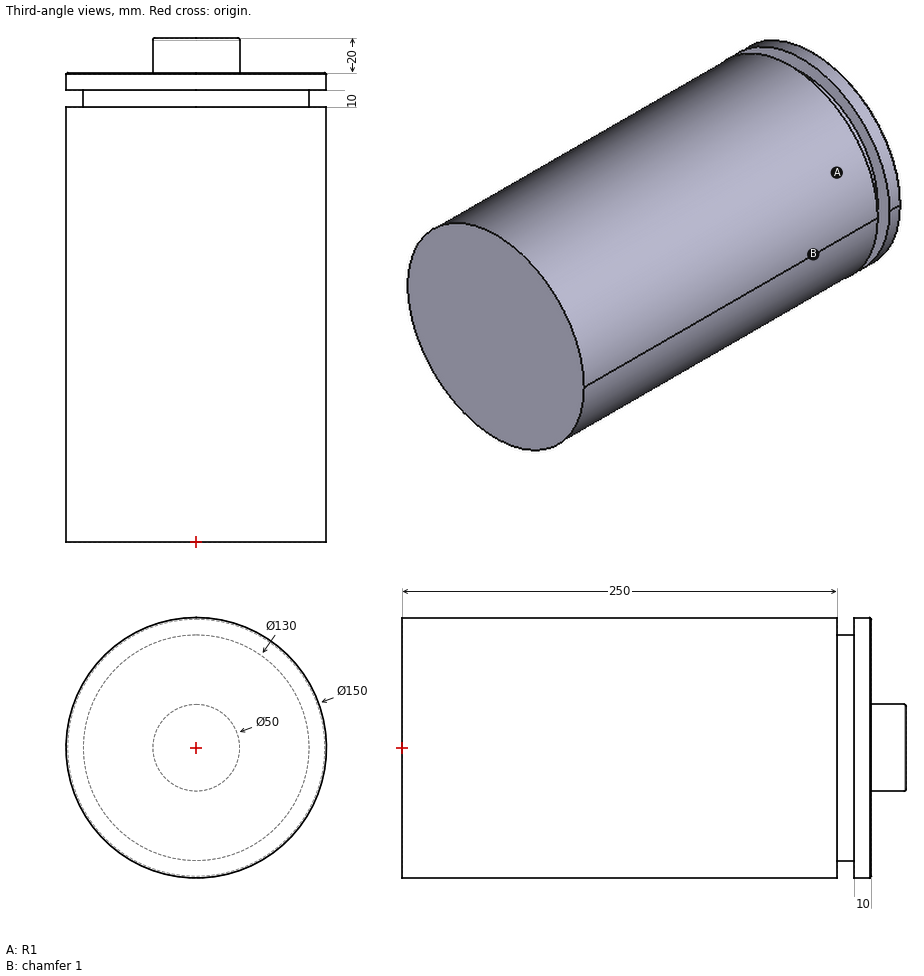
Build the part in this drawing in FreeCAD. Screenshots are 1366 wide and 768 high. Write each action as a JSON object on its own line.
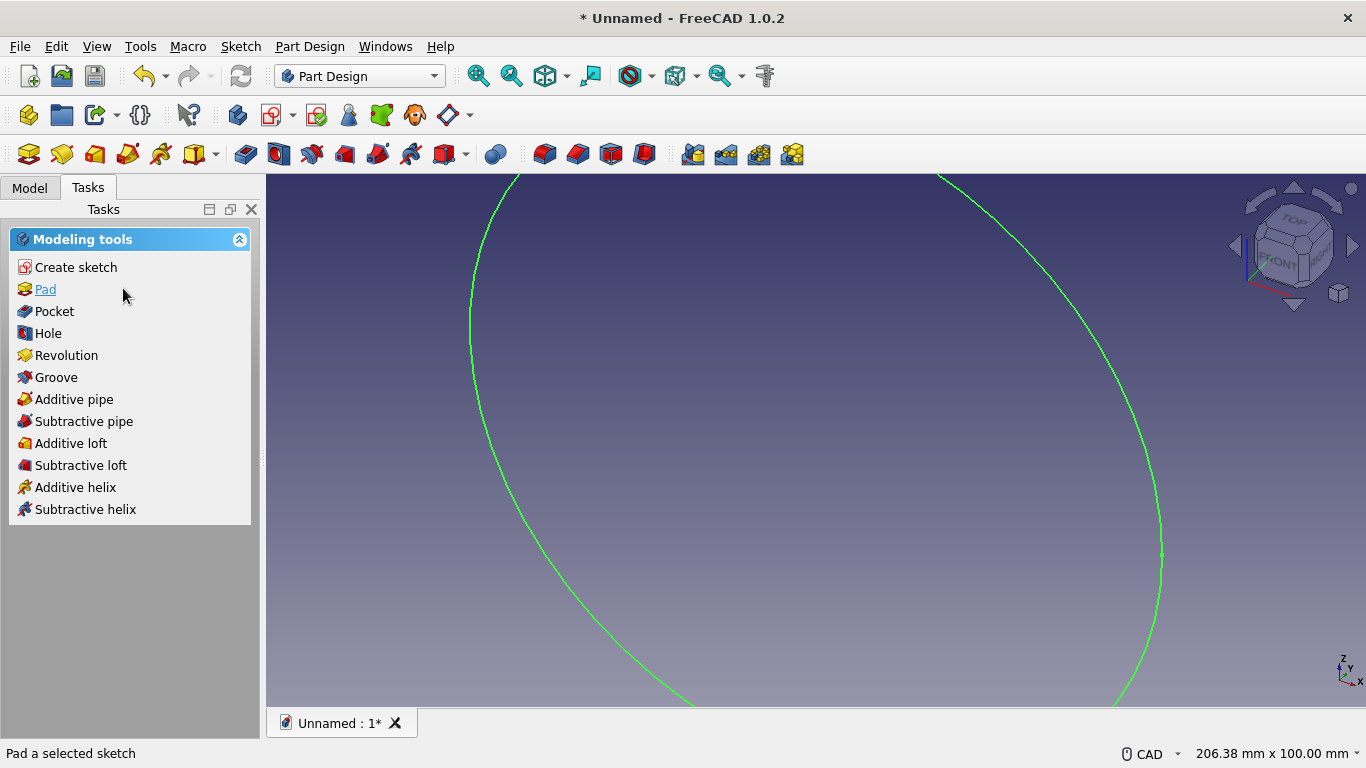
{"action": "left_click", "coordinate": [29, 154]}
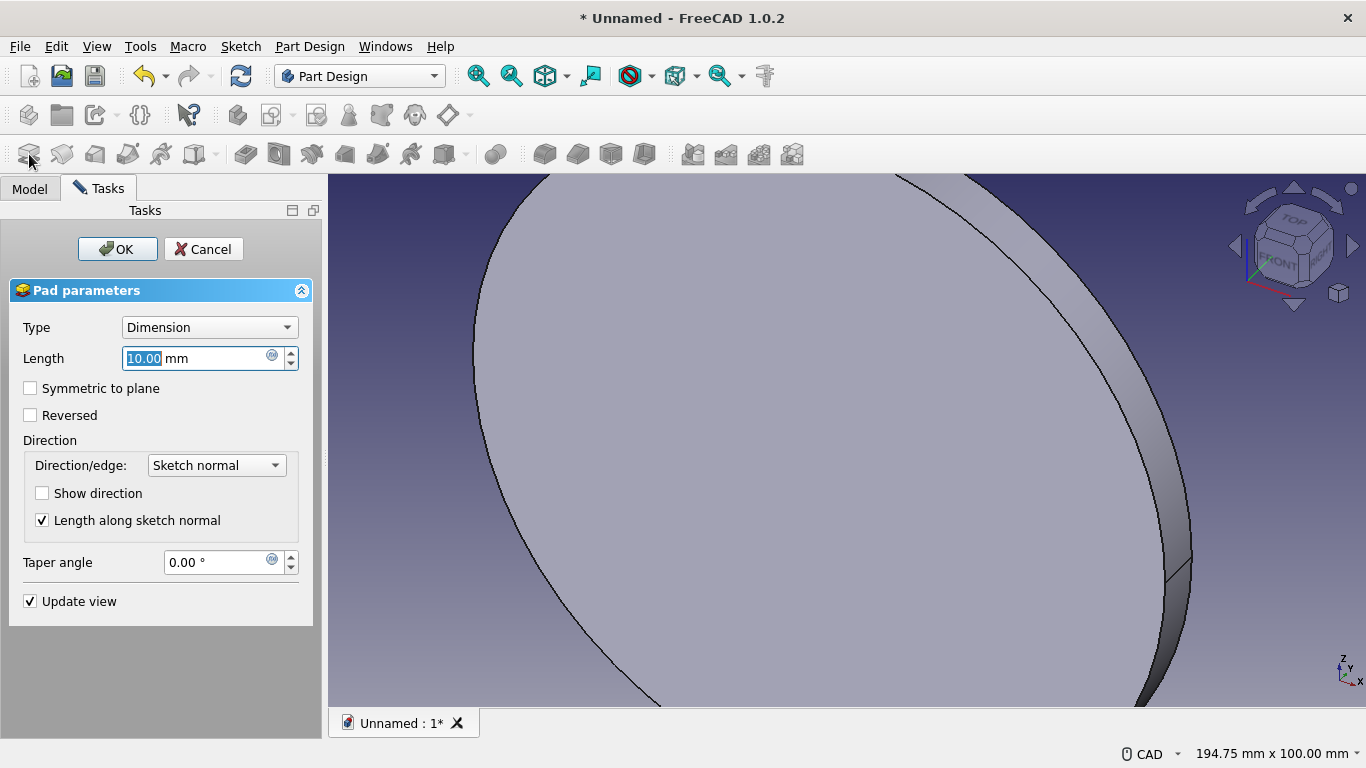
{"action": "type", "text": "250"}
{"action": "key", "text": "Tab"}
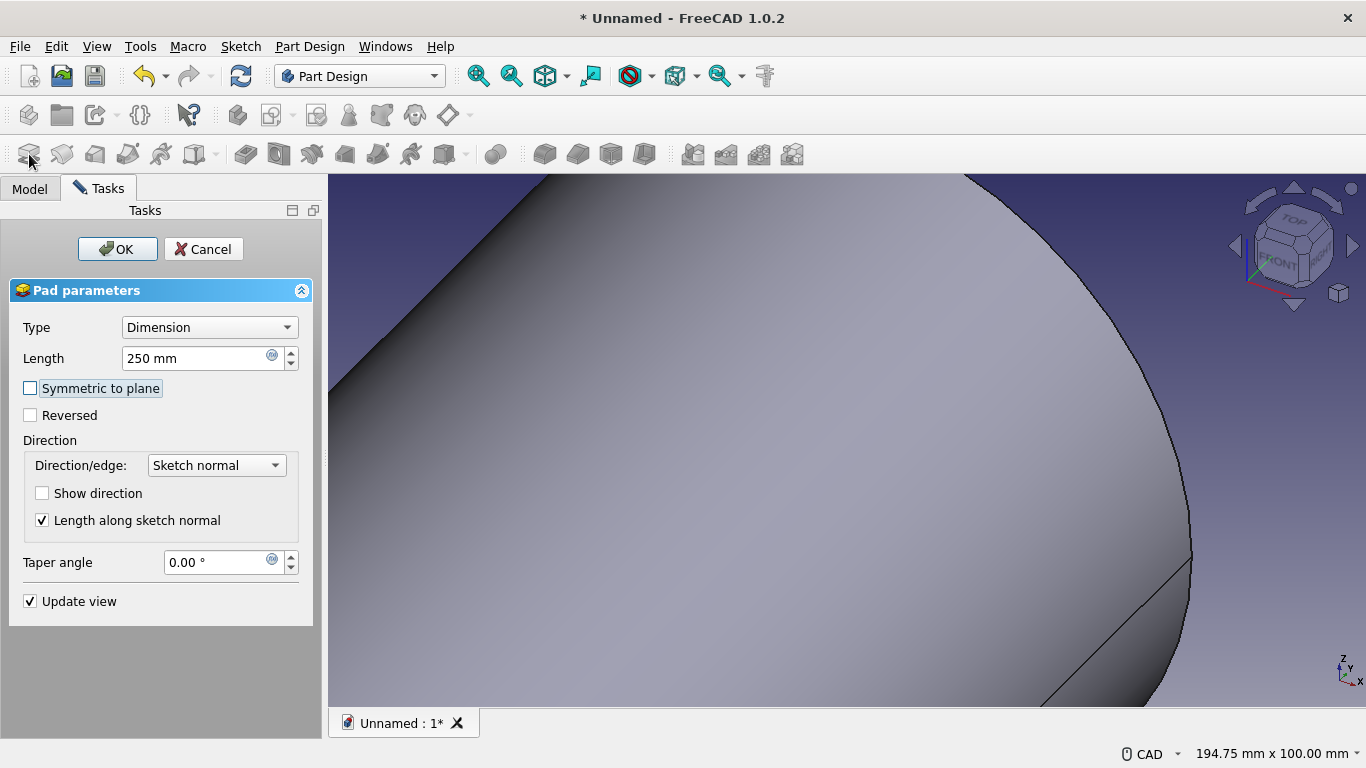
{"action": "left_click", "coordinate": [31, 415]}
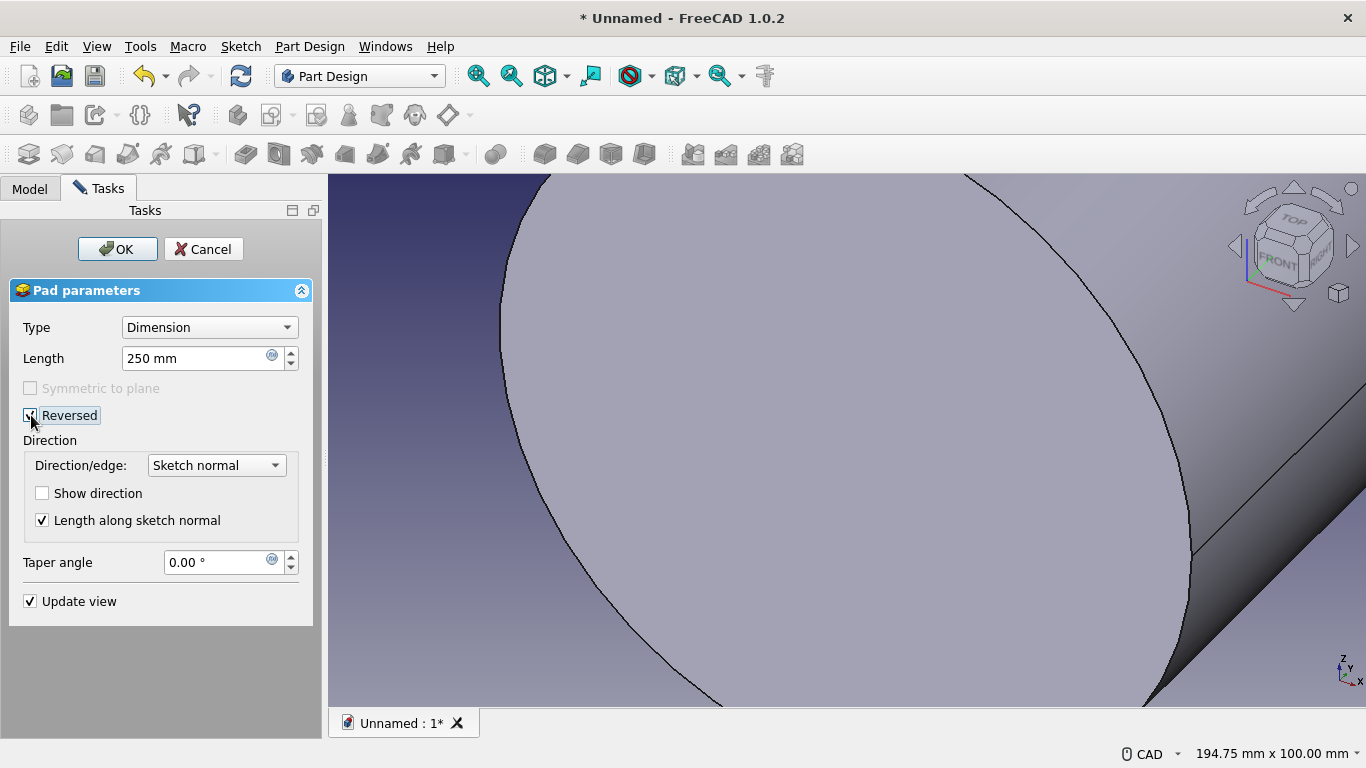
{"action": "left_click", "coordinate": [118, 249]}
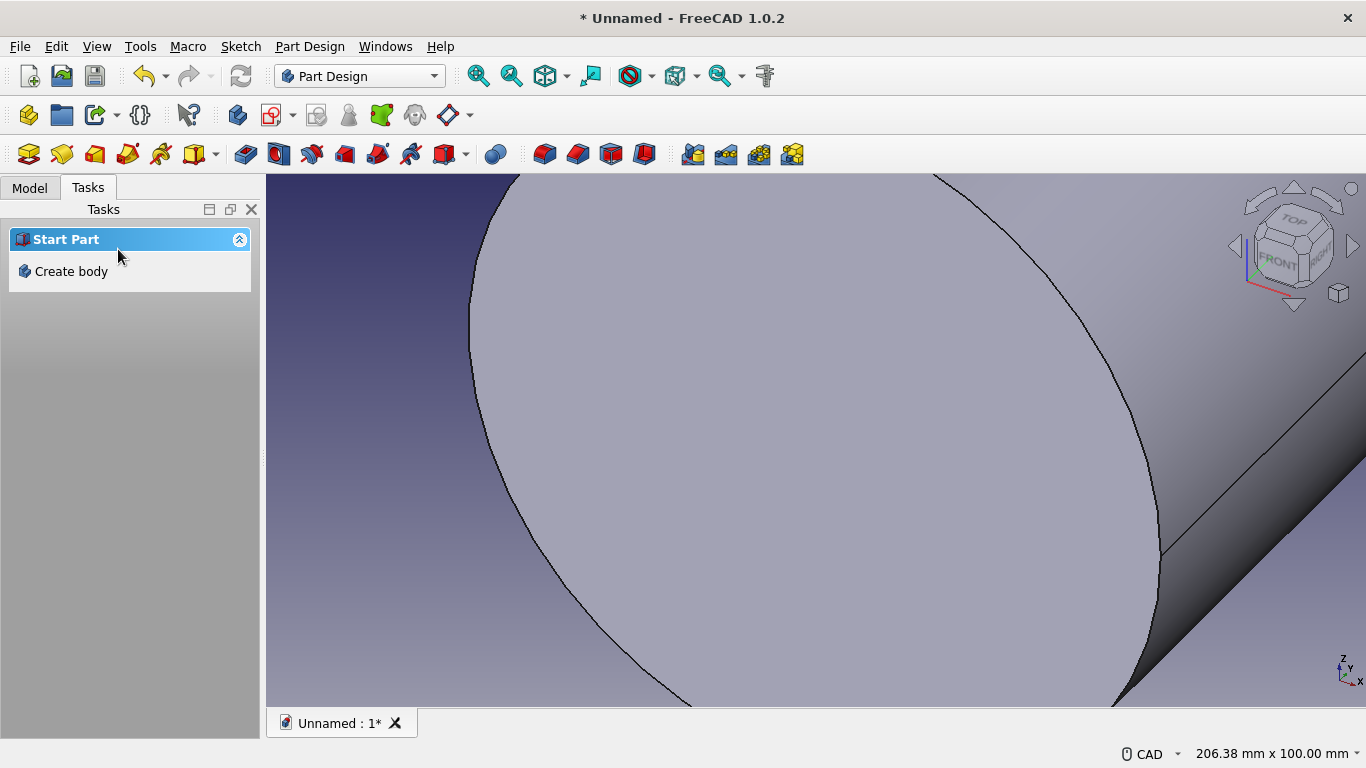
{"action": "key", "text": "v f"}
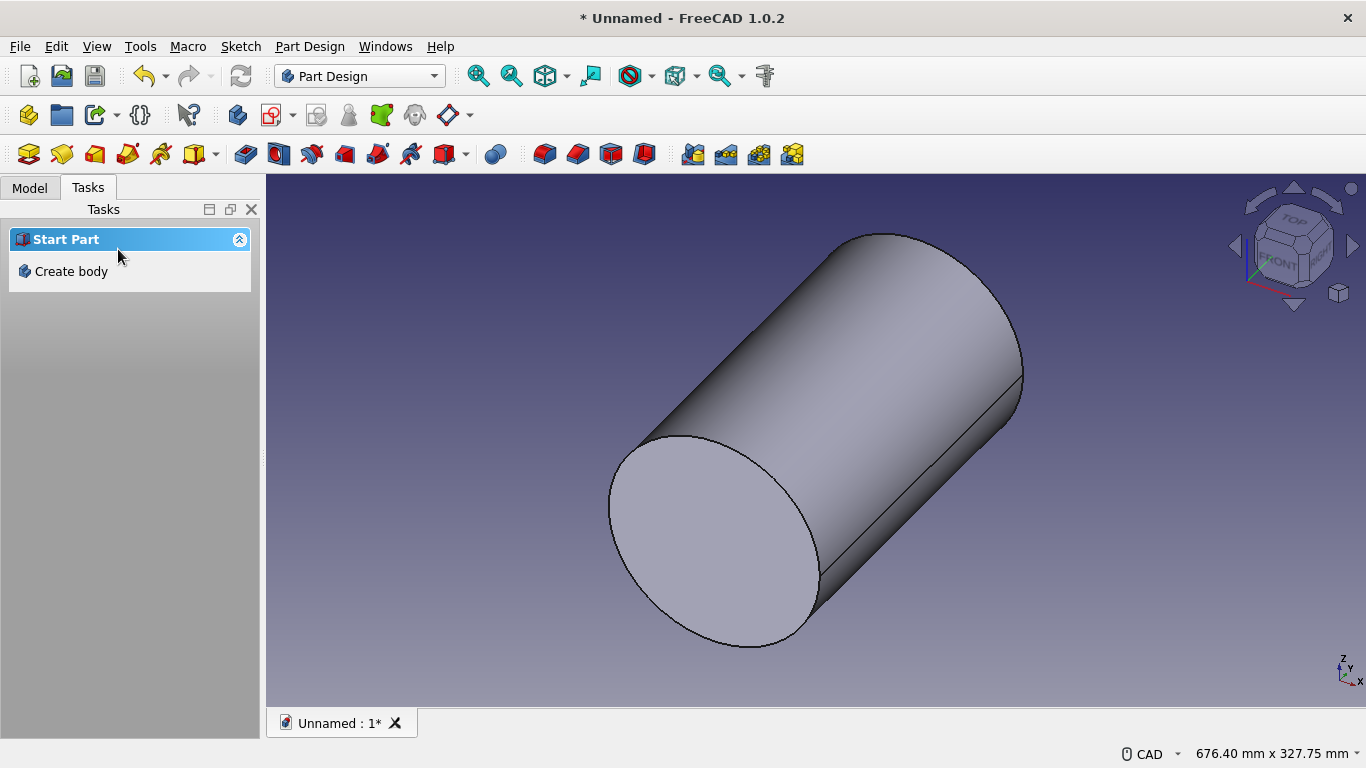
{"action": "key", "text": "4"}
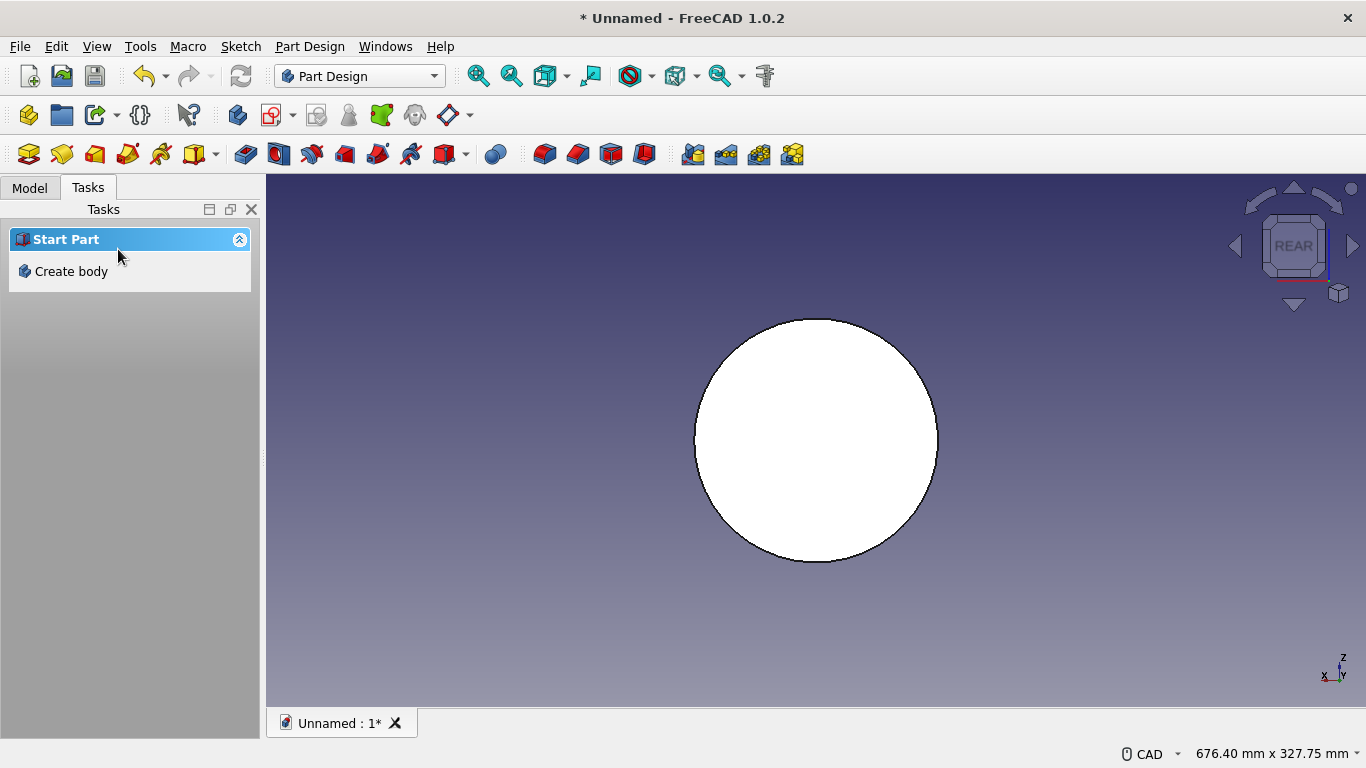
{"action": "left_click", "coordinate": [816, 440]}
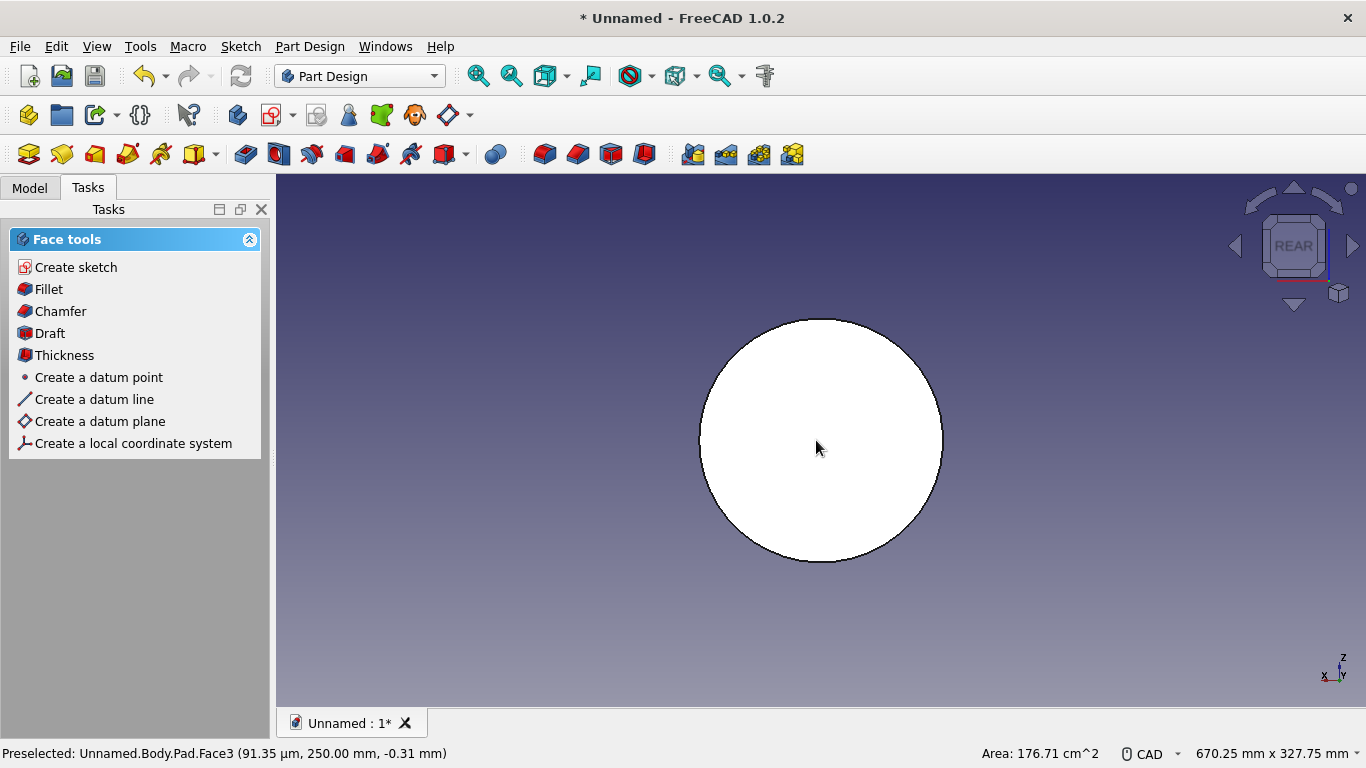
{"action": "left_click", "coordinate": [270, 116]}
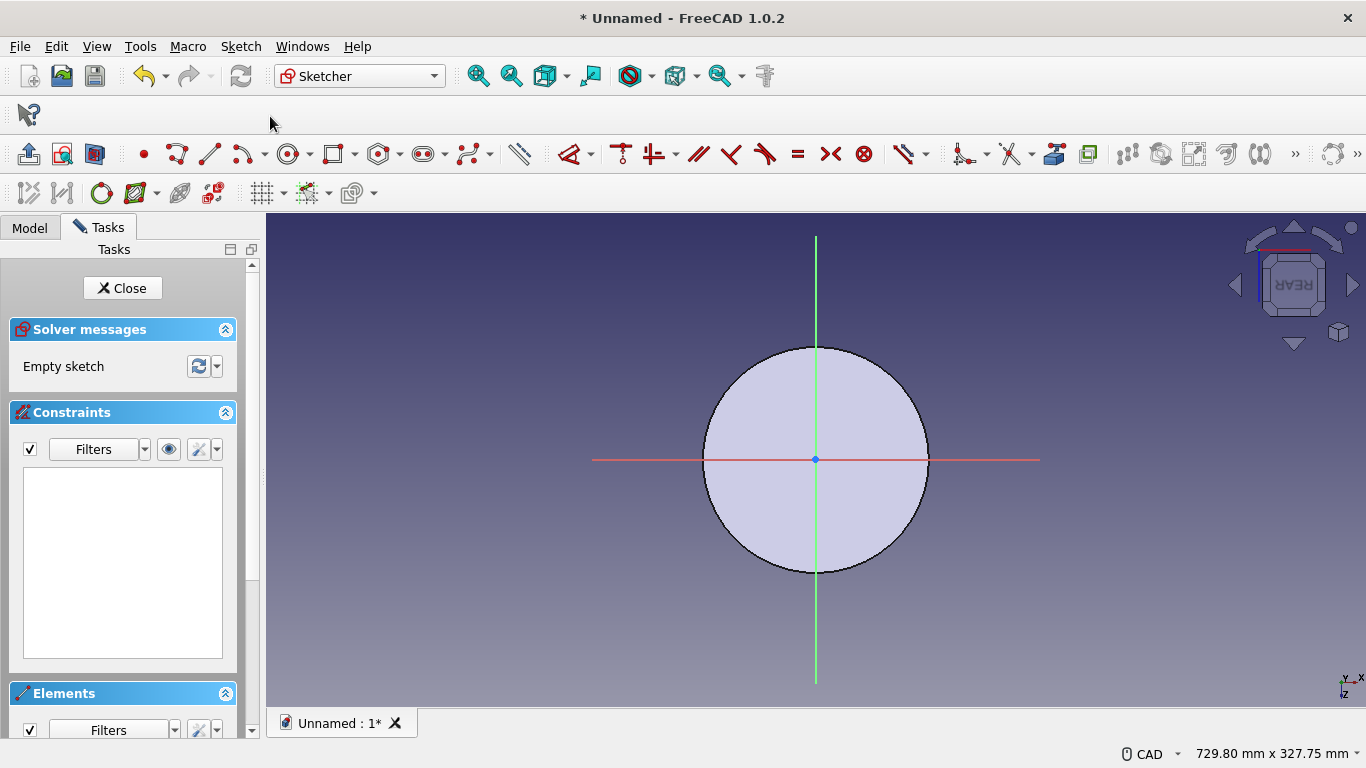
{"action": "scroll", "coordinate": [955, 460], "scroll_direction": "up", "scroll_amount": 2}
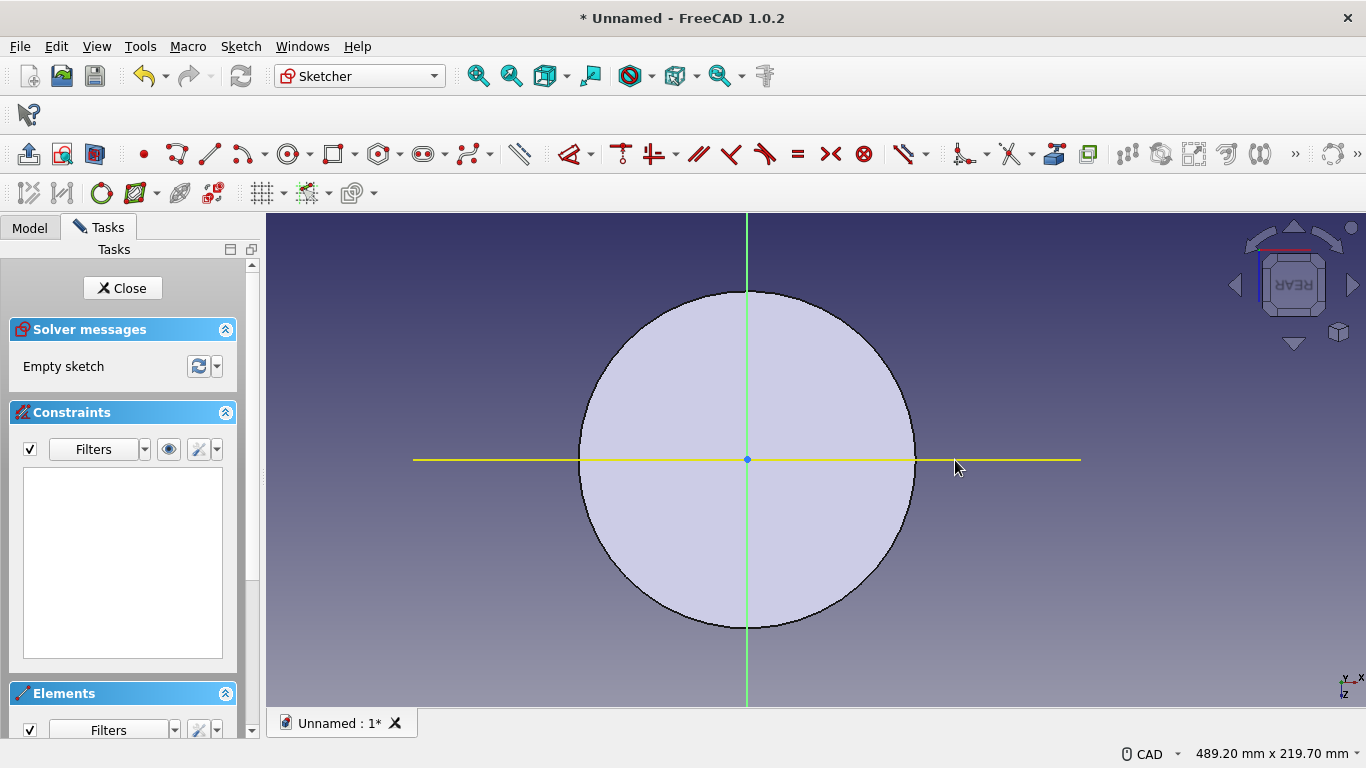
{"action": "key", "text": "g c"}